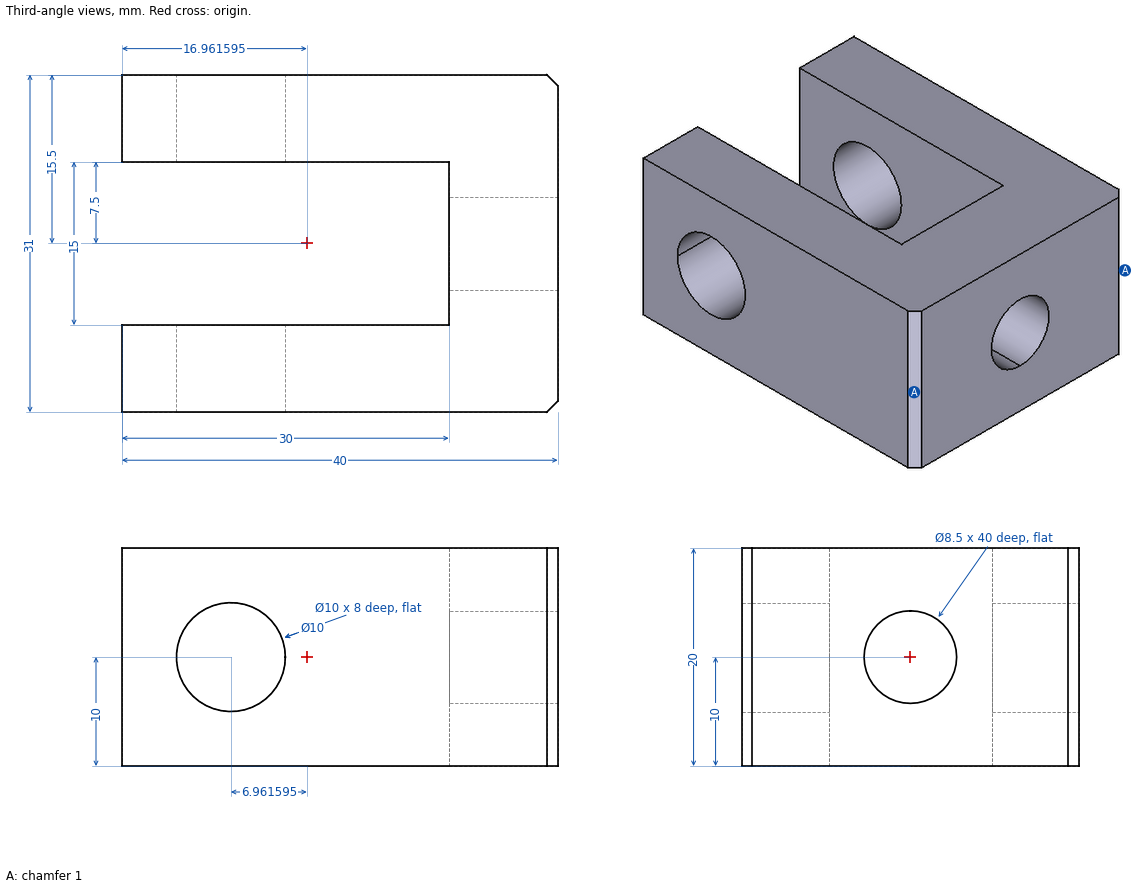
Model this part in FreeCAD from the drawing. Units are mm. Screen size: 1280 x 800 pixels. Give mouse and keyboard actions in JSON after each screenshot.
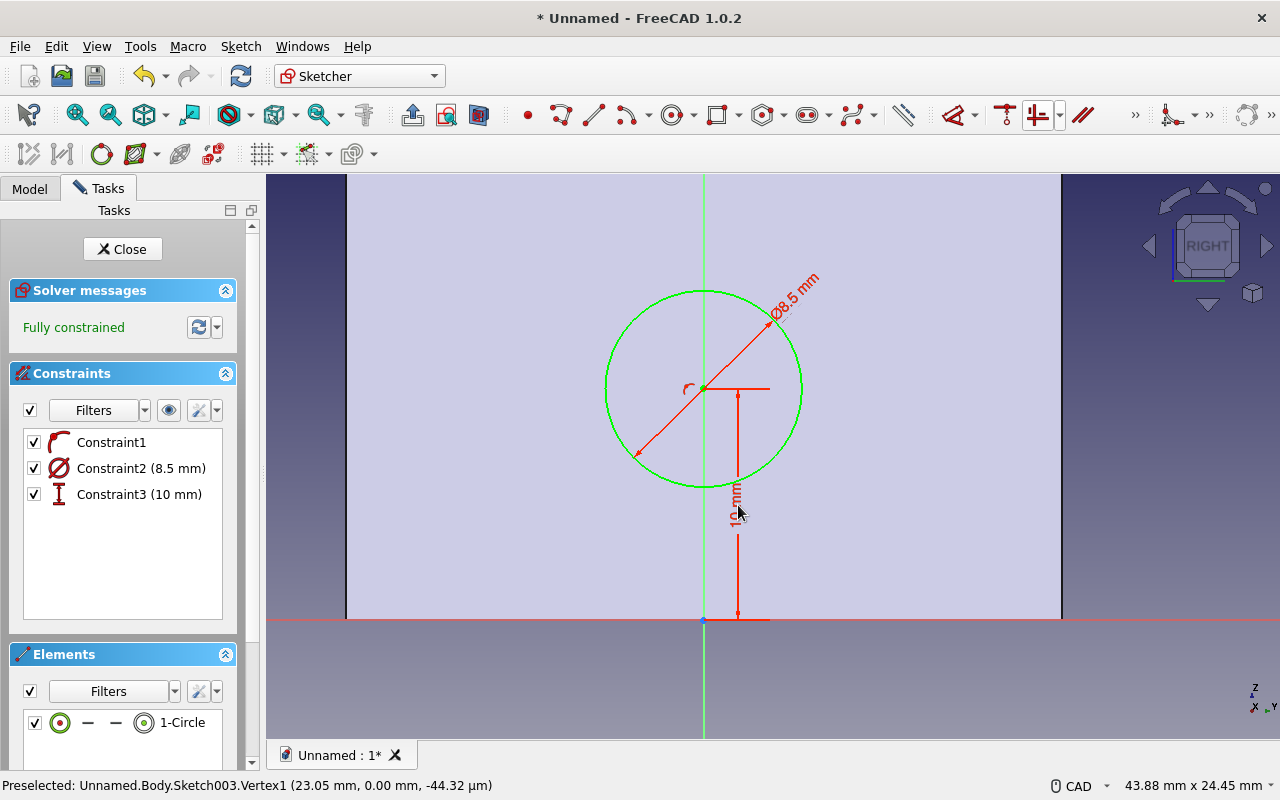
{"action": "left_click", "coordinate": [123, 249]}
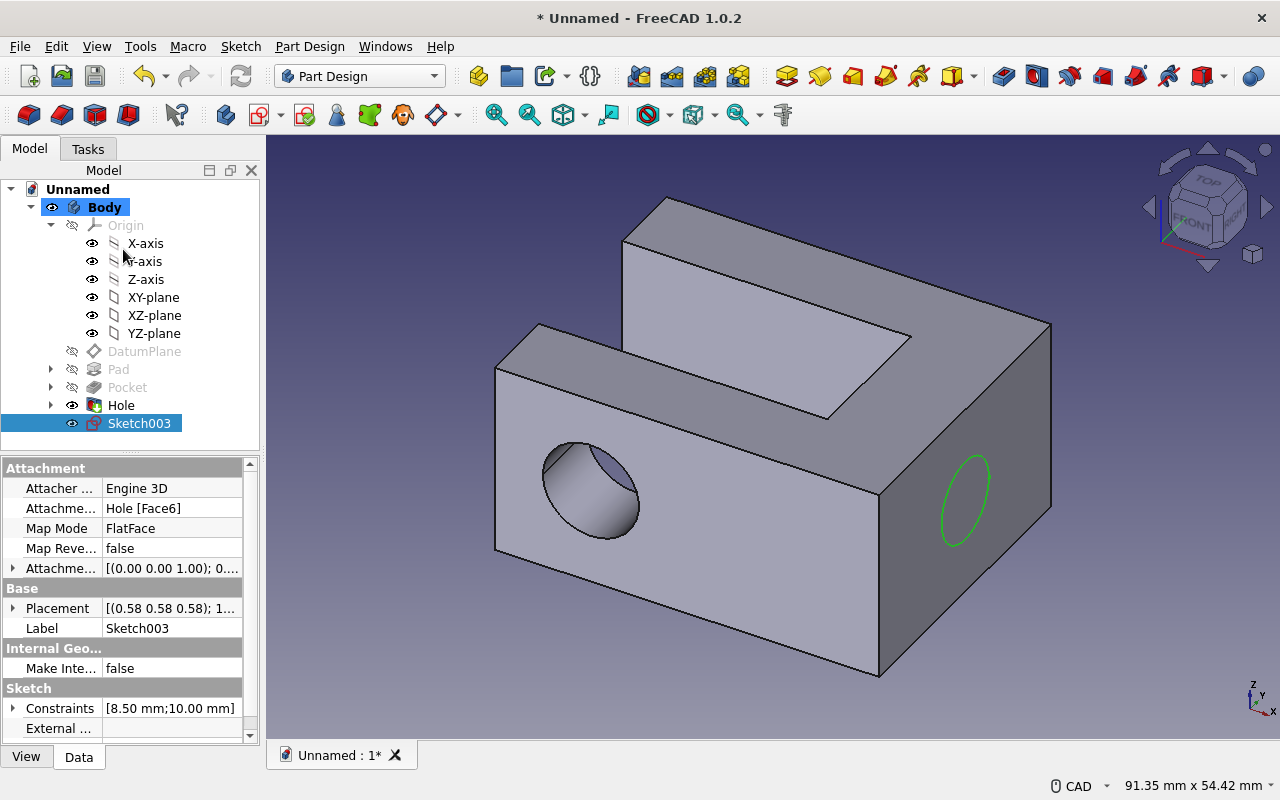
{"action": "left_click", "coordinate": [1037, 76]}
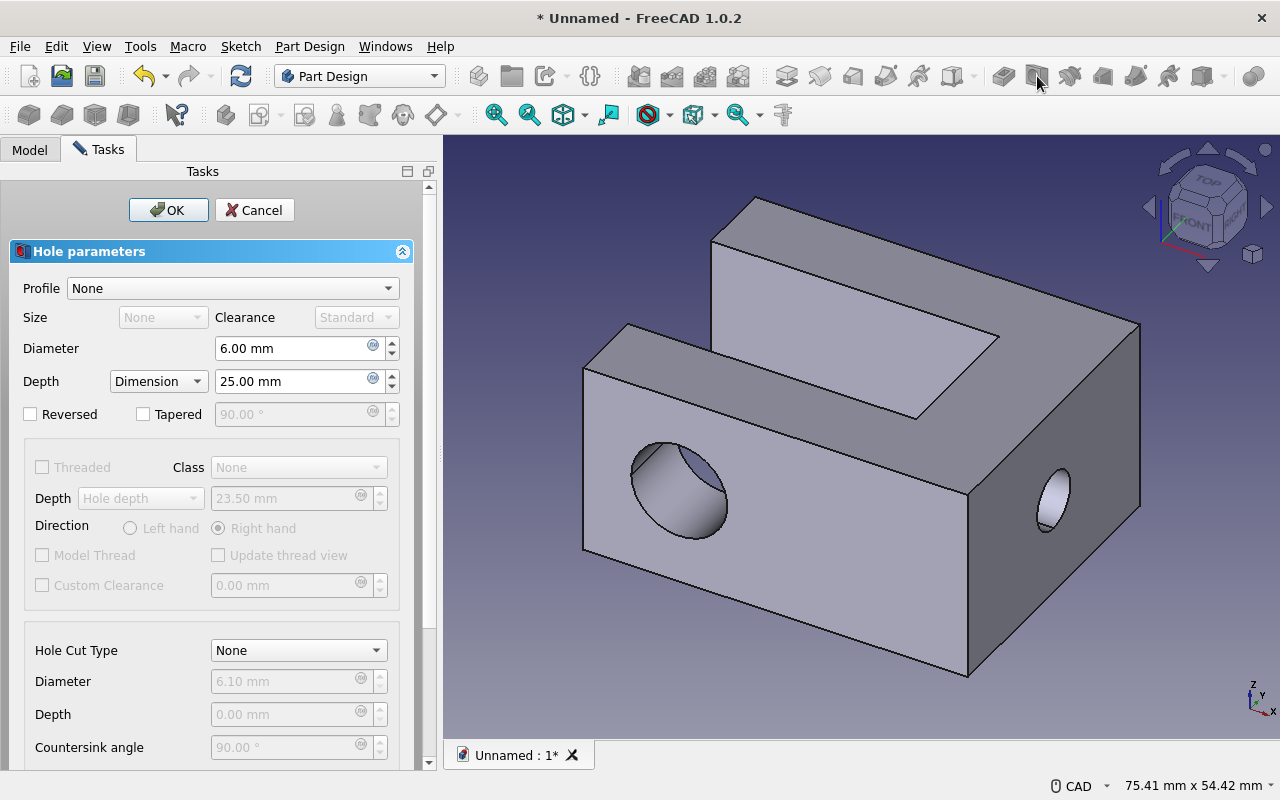
{"action": "triple_click", "coordinate": [300, 348]}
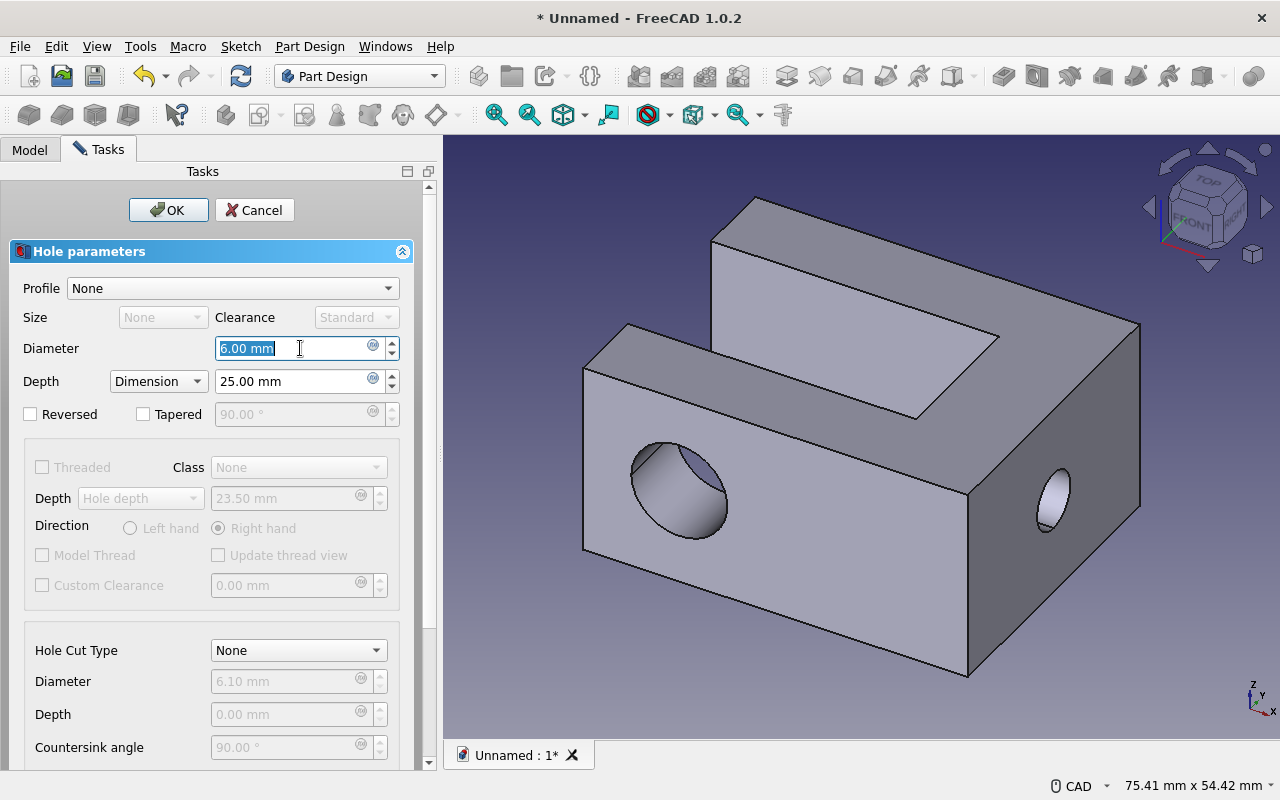
{"action": "type", "text": "8.5"}
{"action": "key", "text": "Tab"}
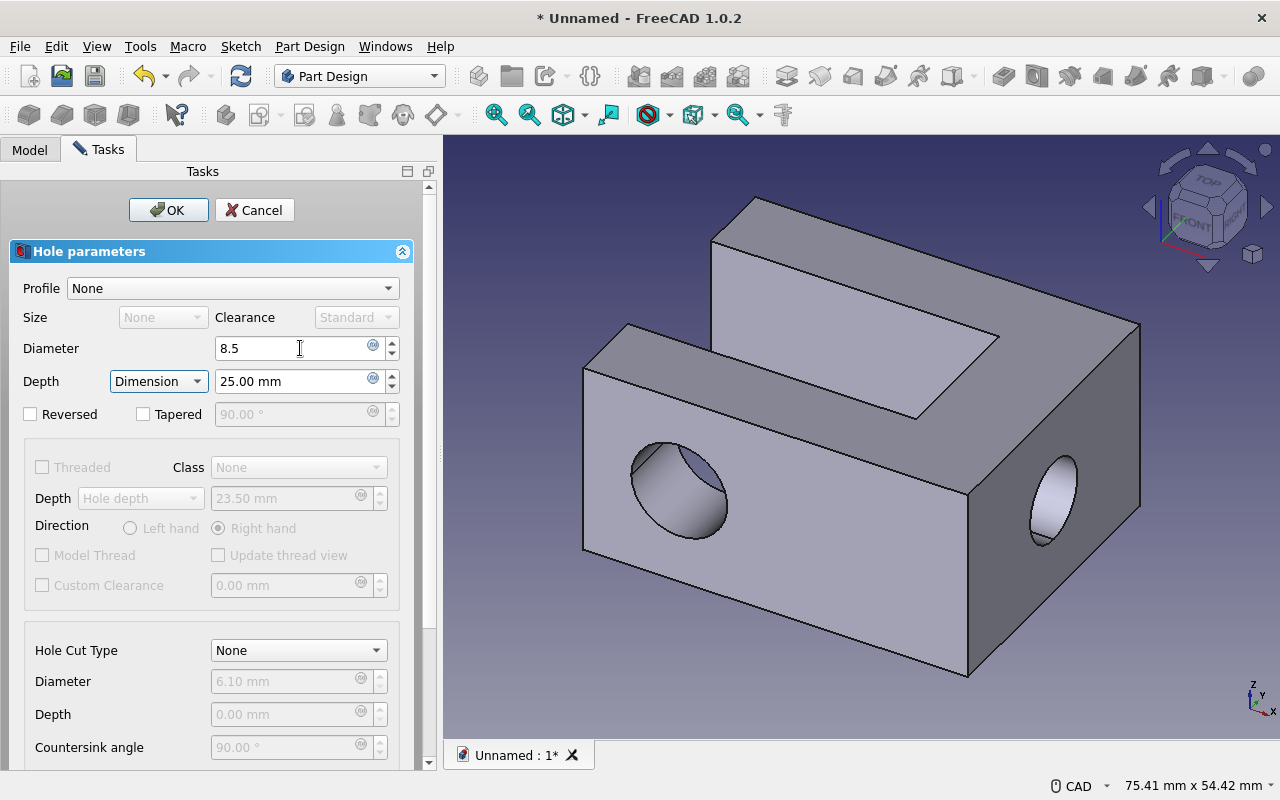
{"action": "triple_click", "coordinate": [300, 382]}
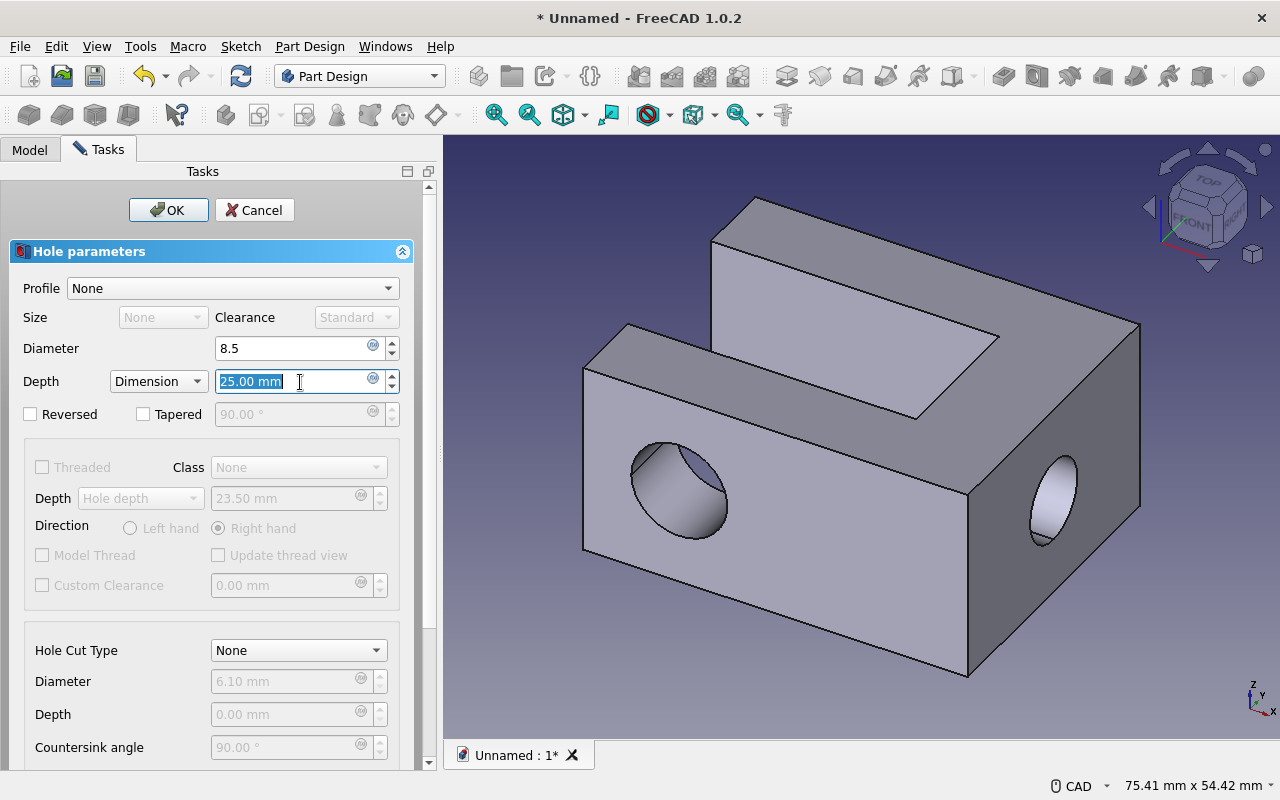
{"action": "type", "text": "40"}
{"action": "key", "text": "Tab"}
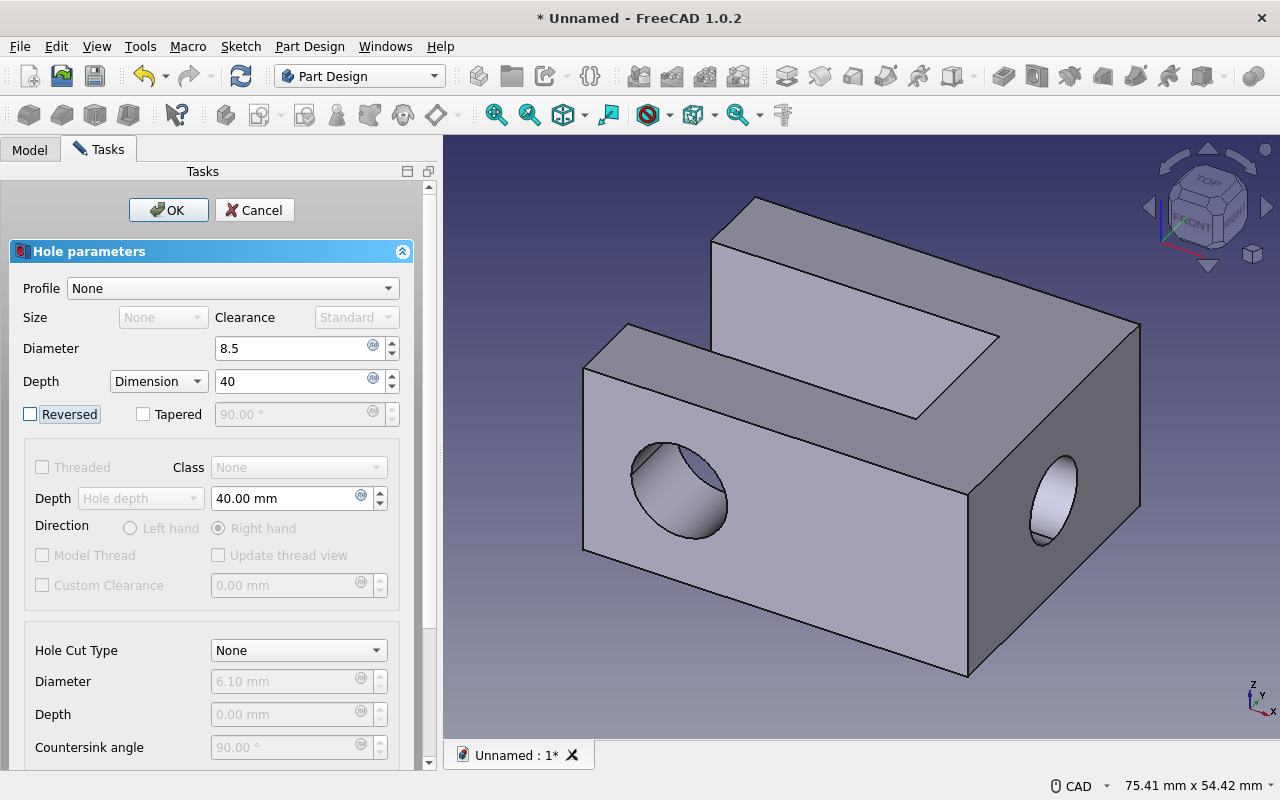
{"action": "scroll", "coordinate": [429, 476], "scroll_direction": "down", "scroll_amount": 3}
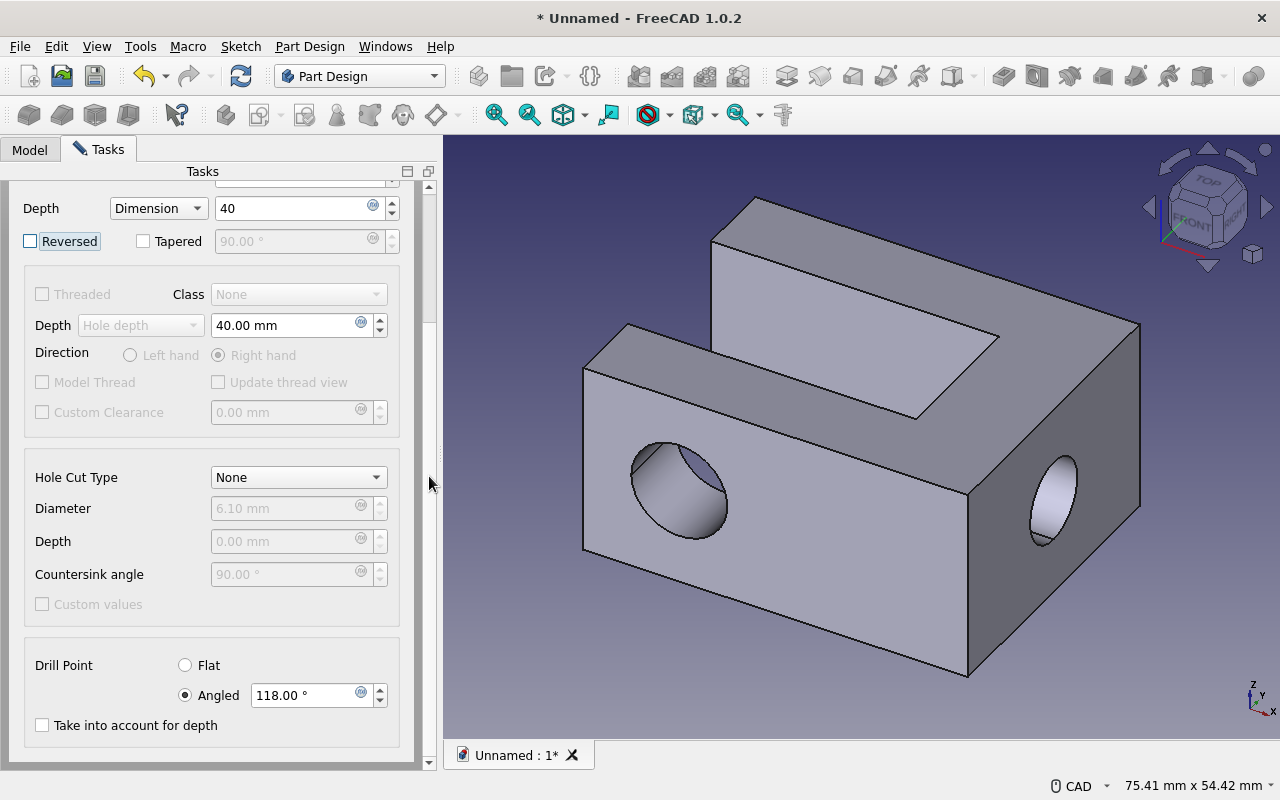
{"action": "left_click", "coordinate": [186, 663]}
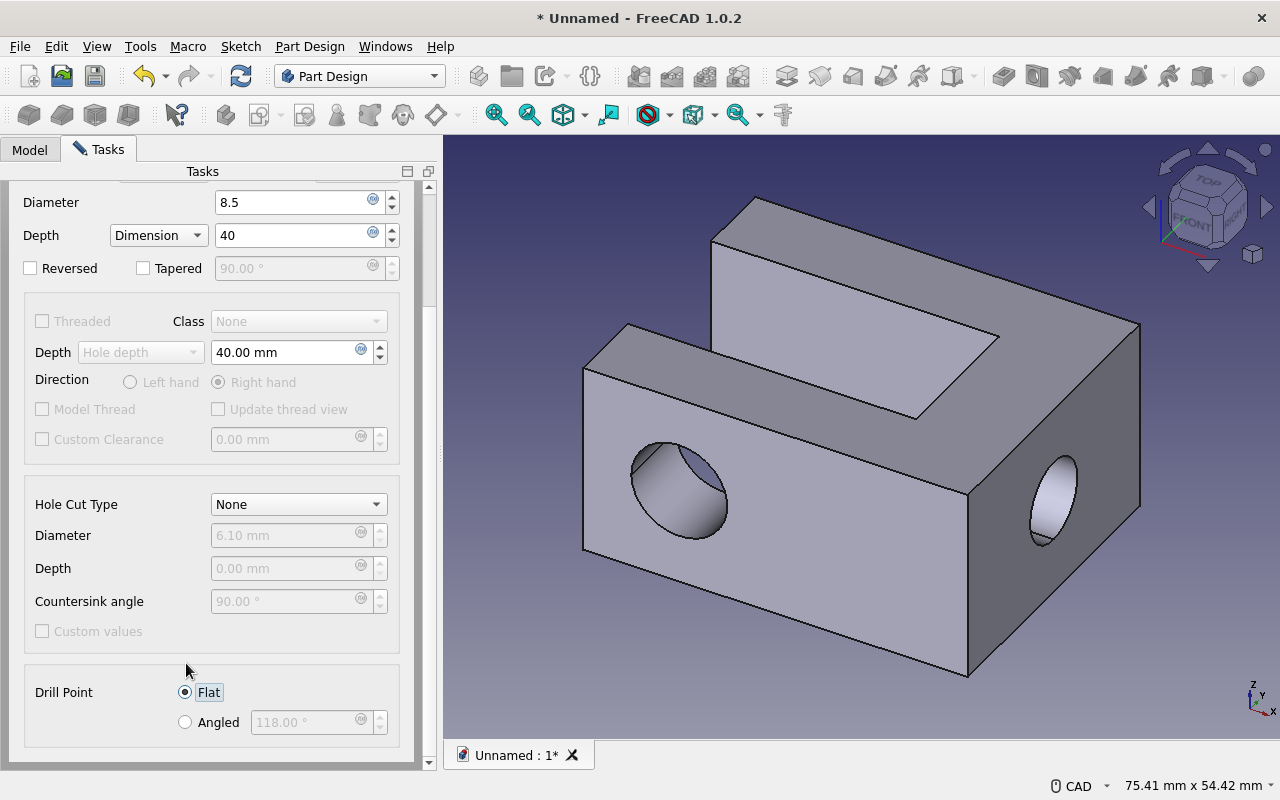
{"action": "scroll", "coordinate": [429, 476], "scroll_direction": "up", "scroll_amount": 4}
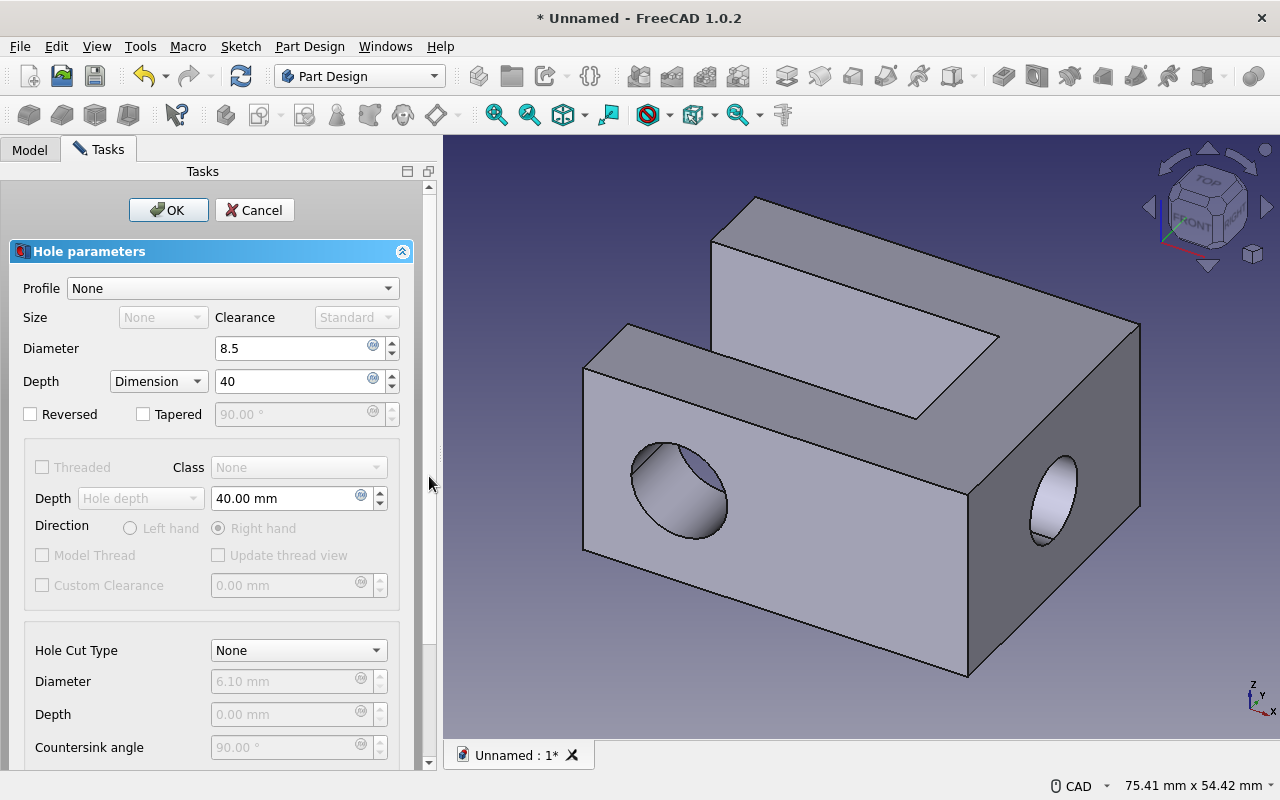
{"action": "left_click", "coordinate": [169, 210]}